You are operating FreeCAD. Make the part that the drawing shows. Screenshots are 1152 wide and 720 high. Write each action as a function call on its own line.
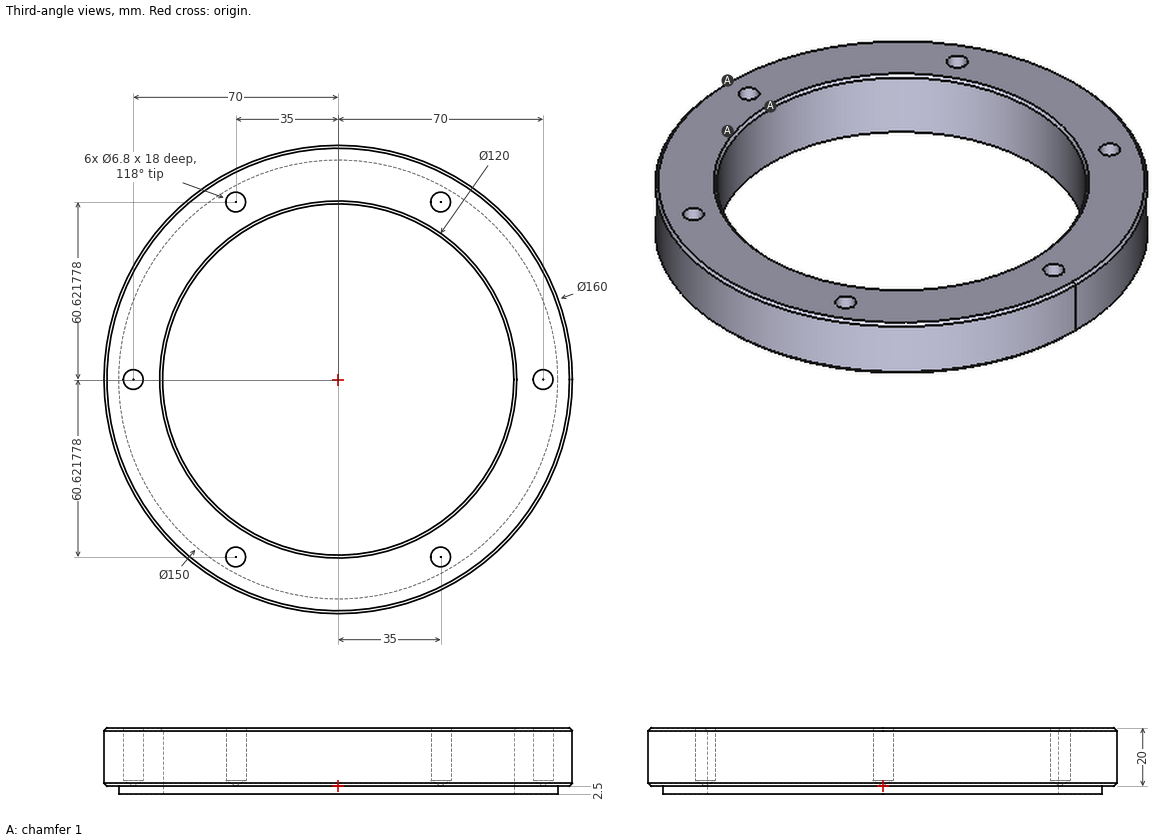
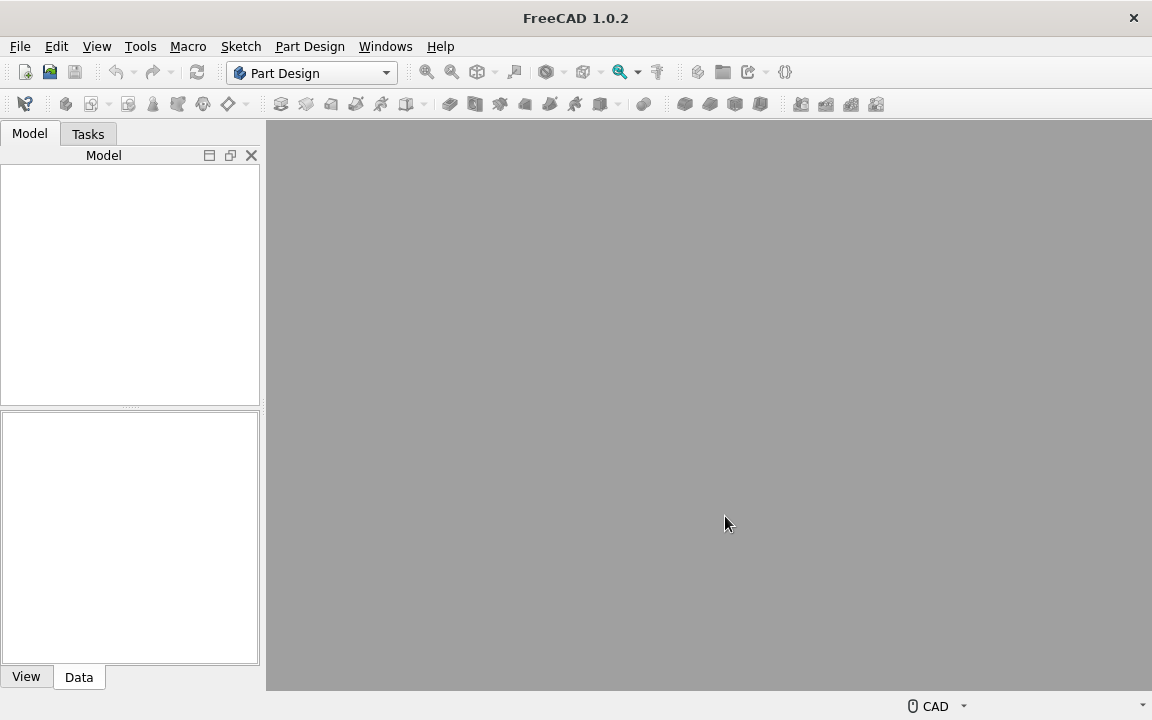
click(25, 72)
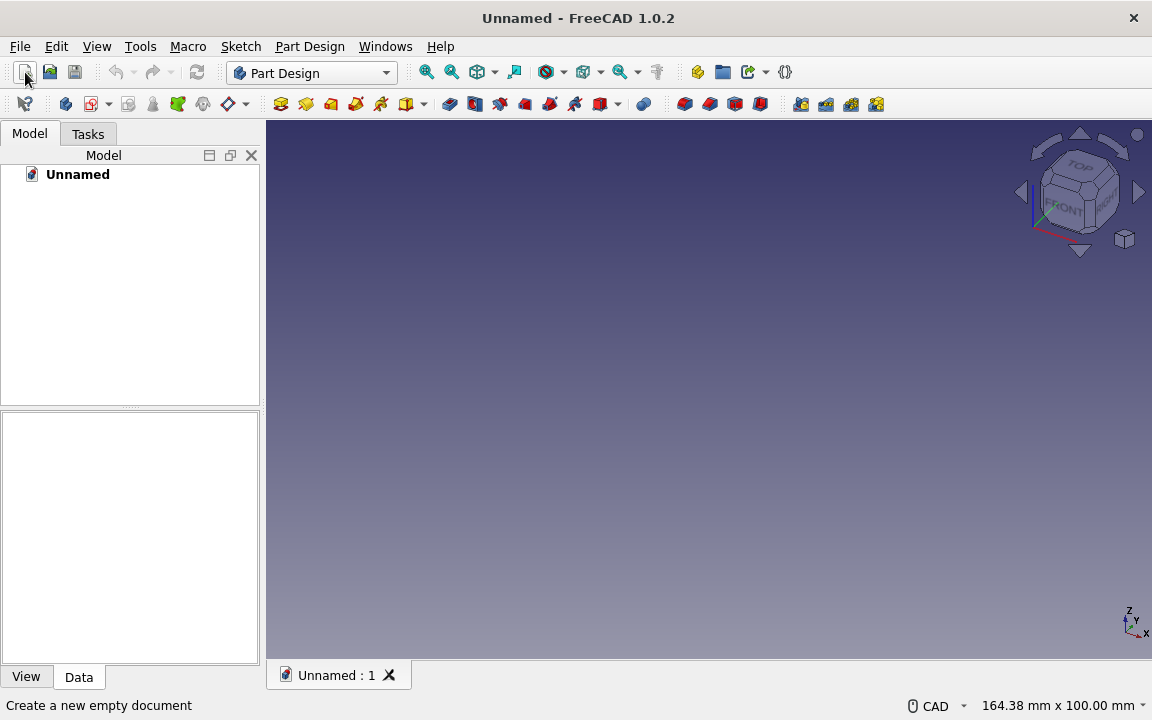
click(90, 104)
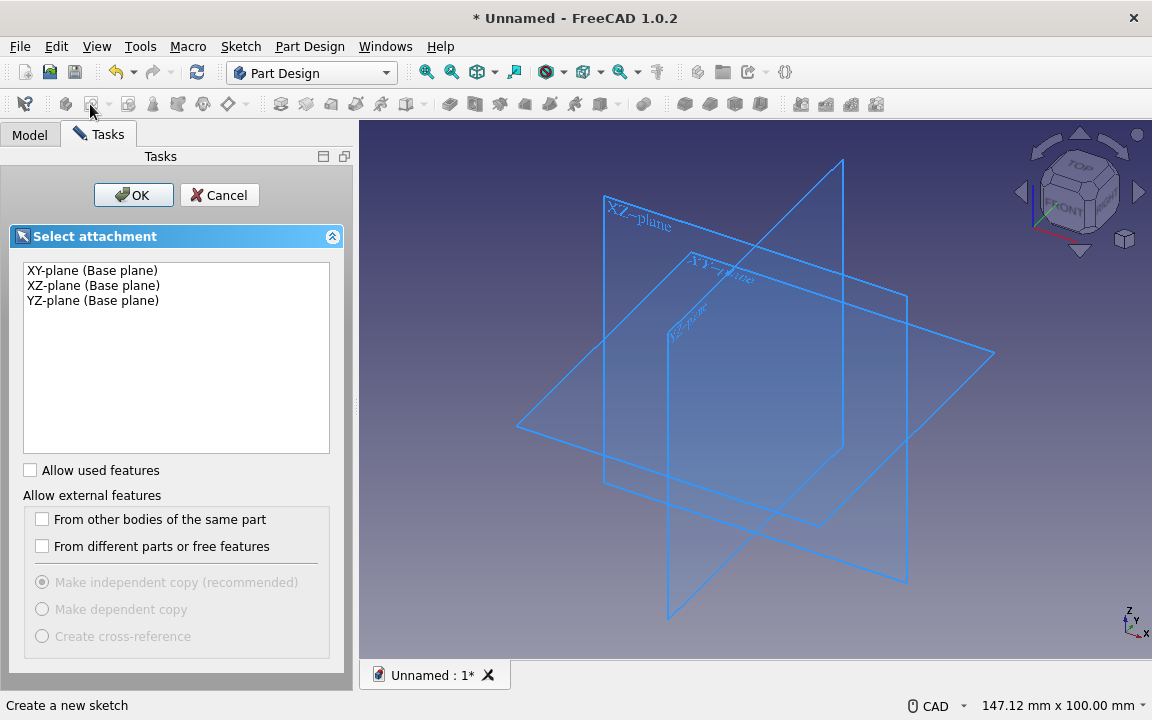
click(84, 270)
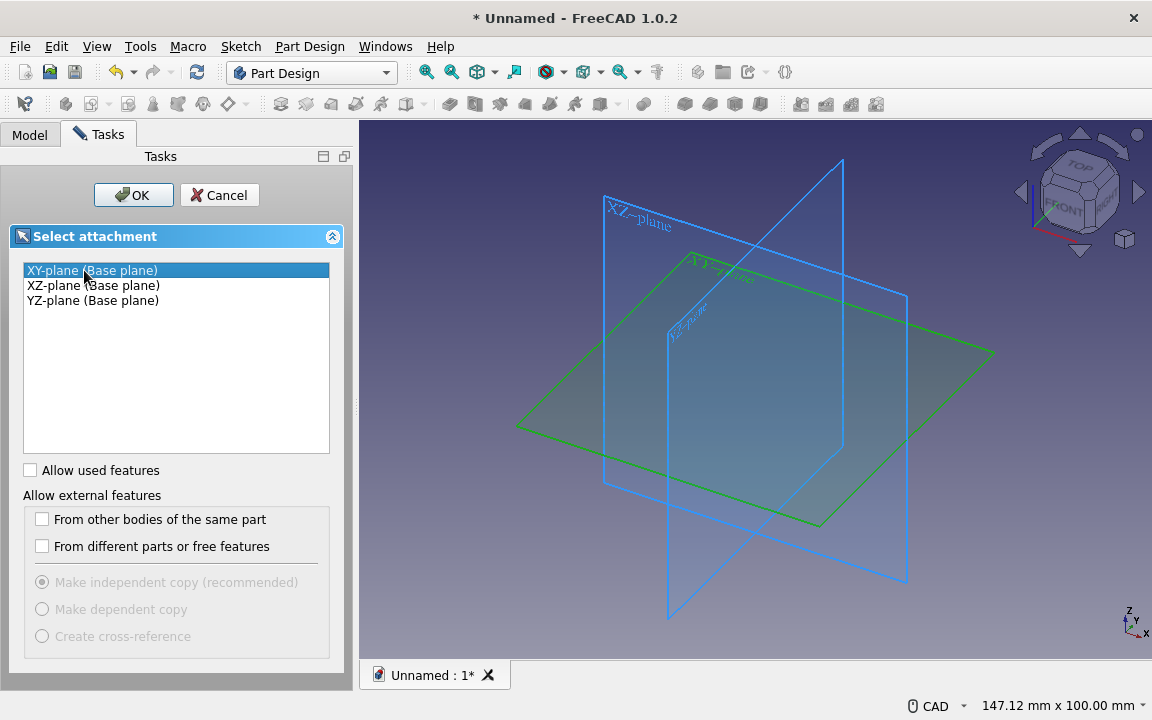
click(134, 195)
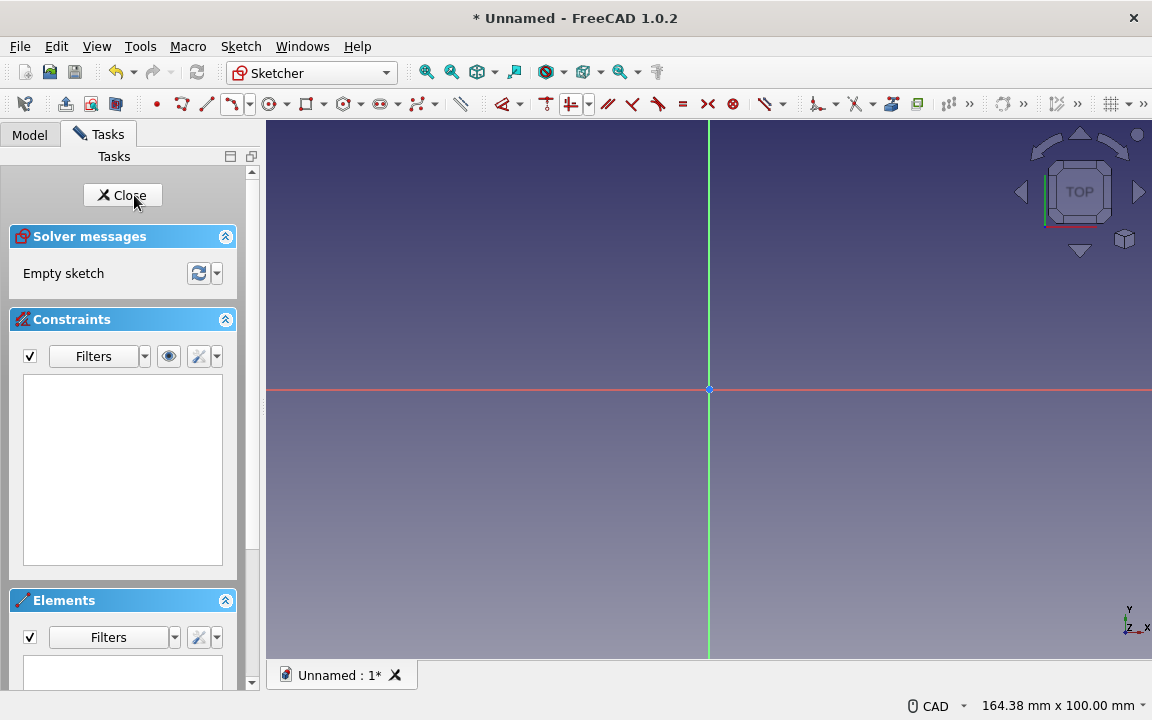
scroll(601, 390, down, 5)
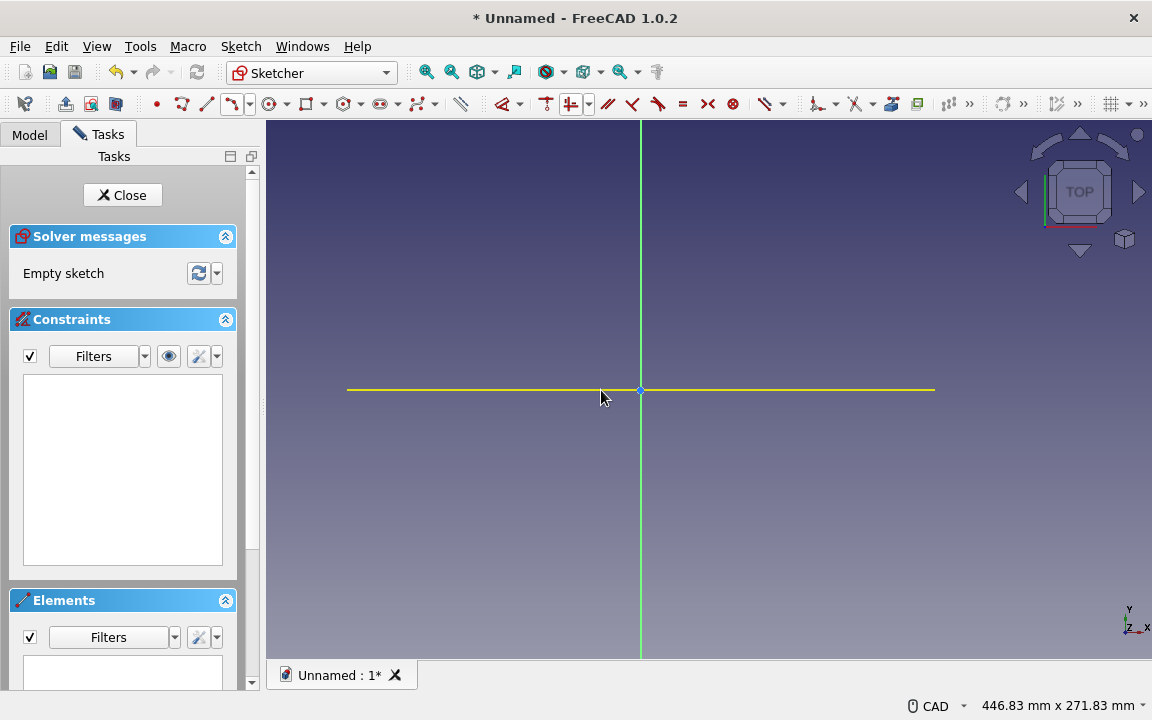
click(268, 104)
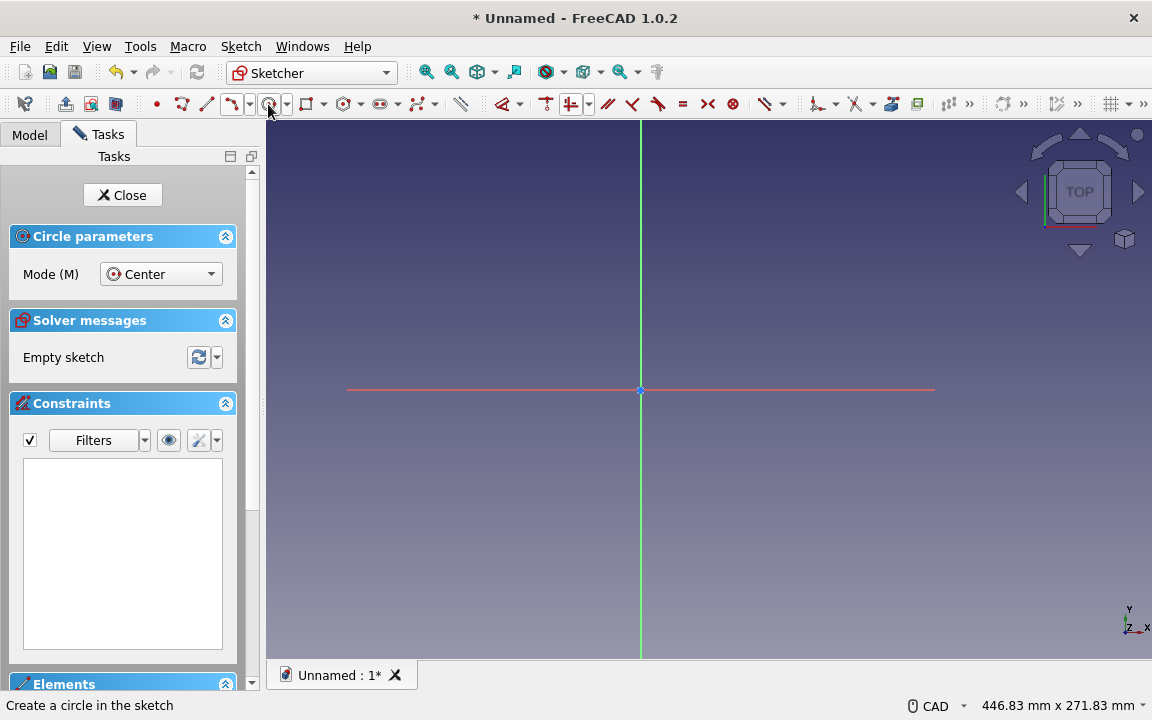
click(641, 390)
click(753, 278)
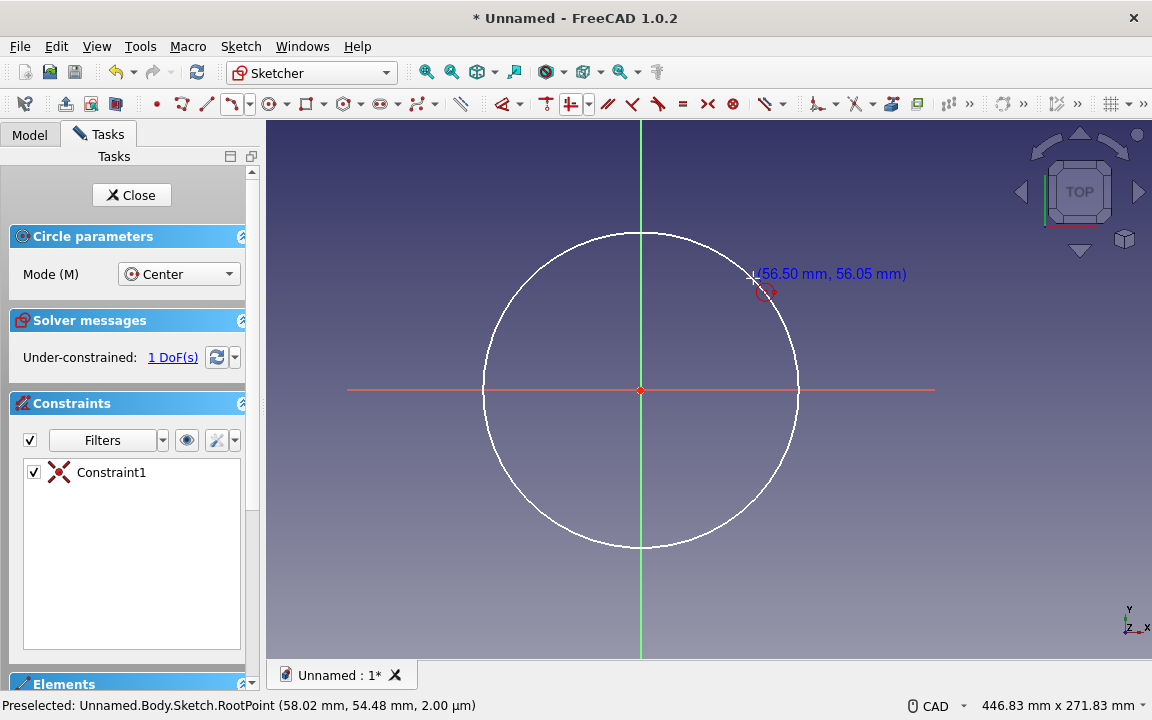
click(641, 390)
click(725, 306)
key(Escape)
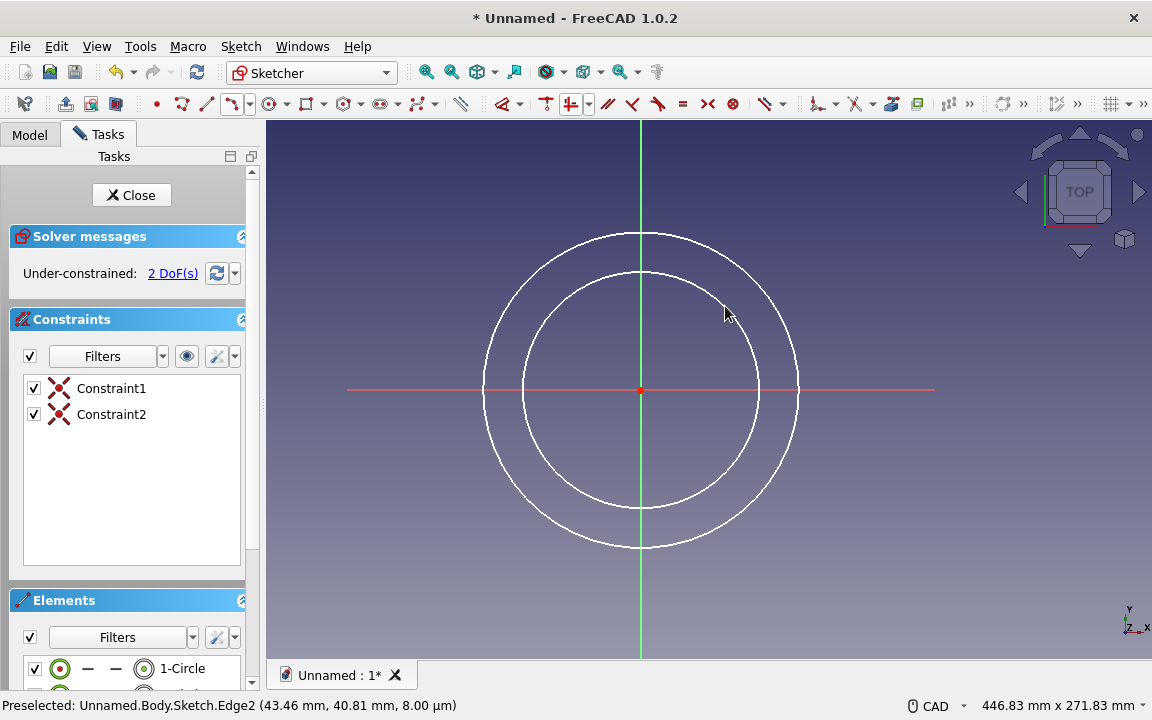
click(502, 104)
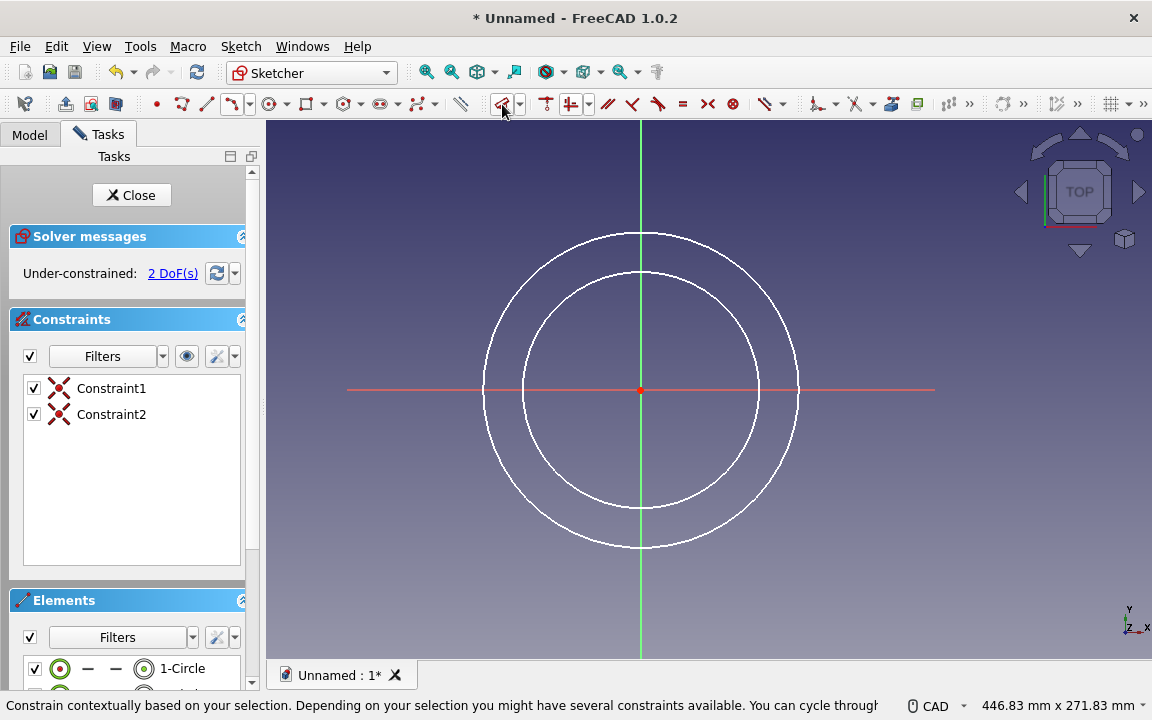
click(752, 278)
click(775, 255)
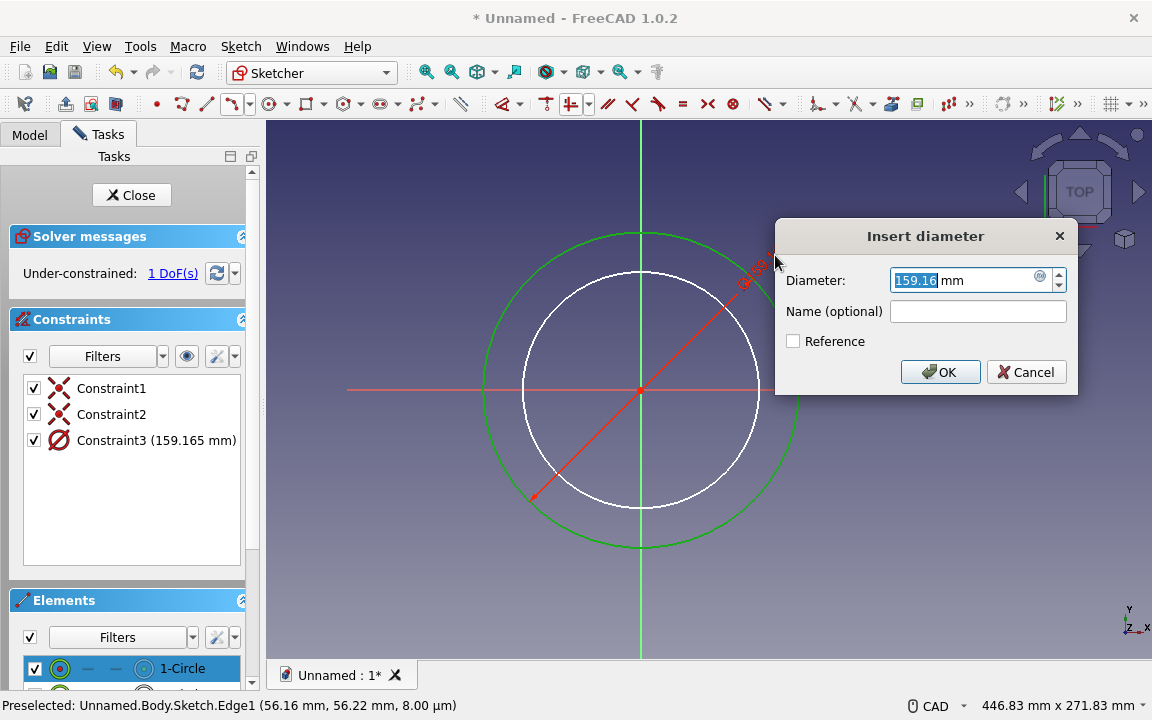
text(160)
key(Return)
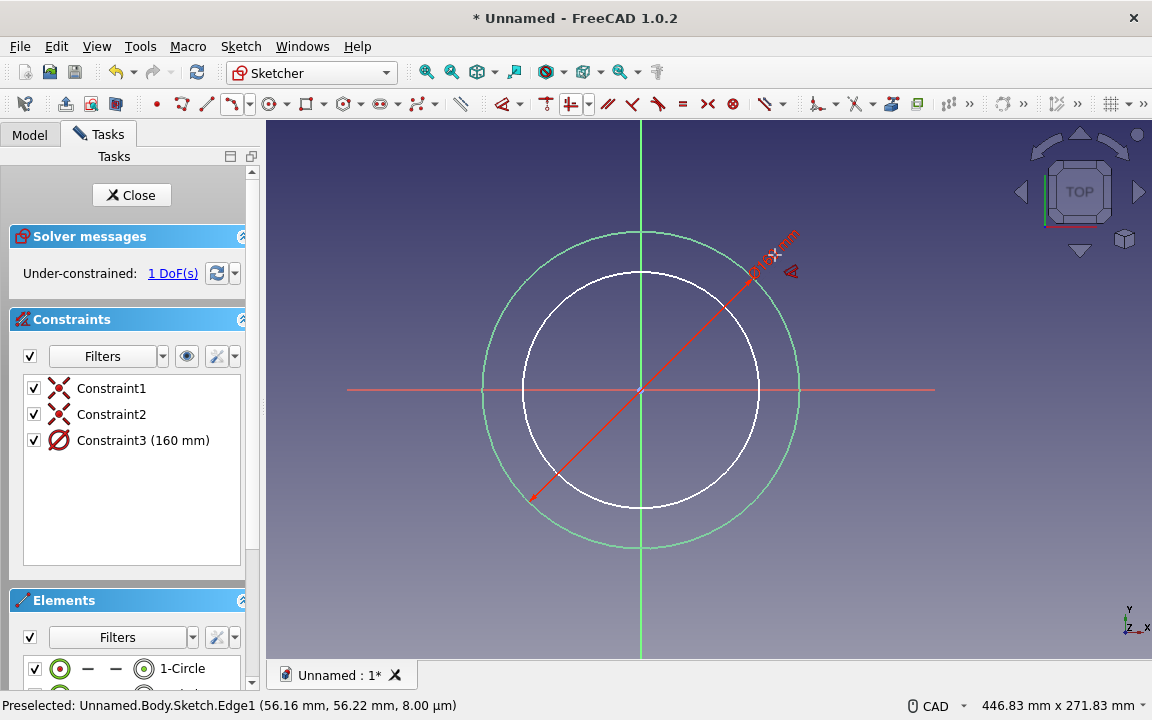
click(724, 306)
click(807, 340)